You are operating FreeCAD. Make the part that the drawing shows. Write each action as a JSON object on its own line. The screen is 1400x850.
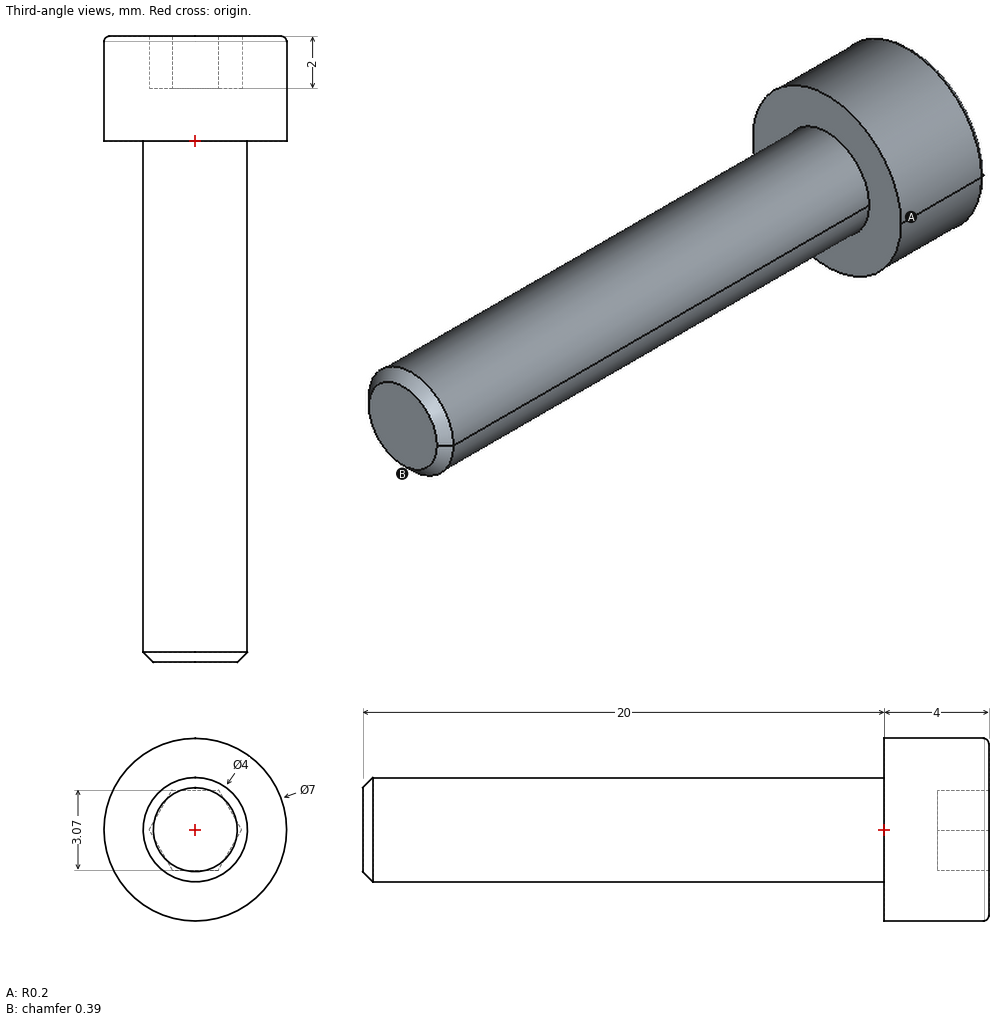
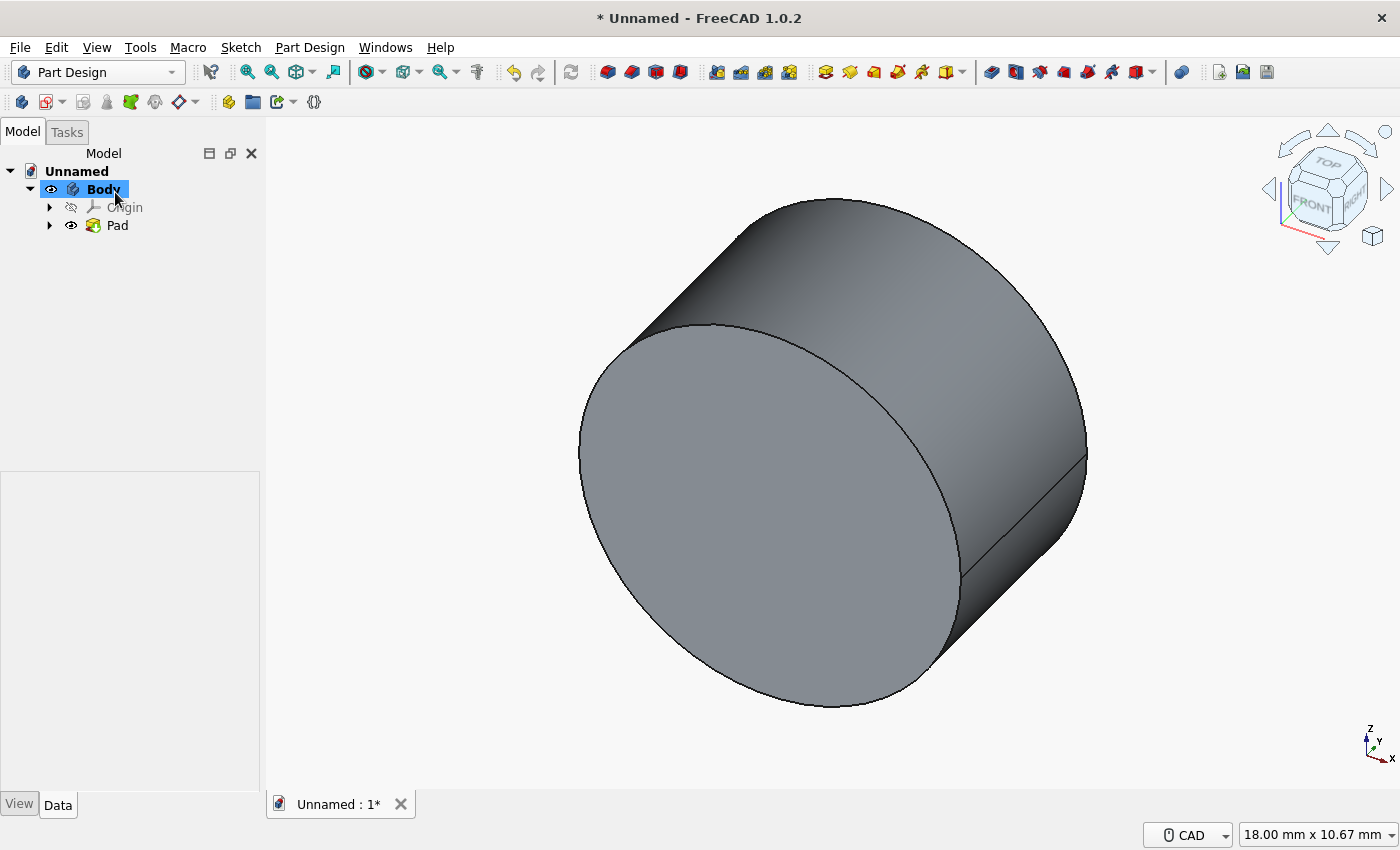
{"action": "key", "text": "4"}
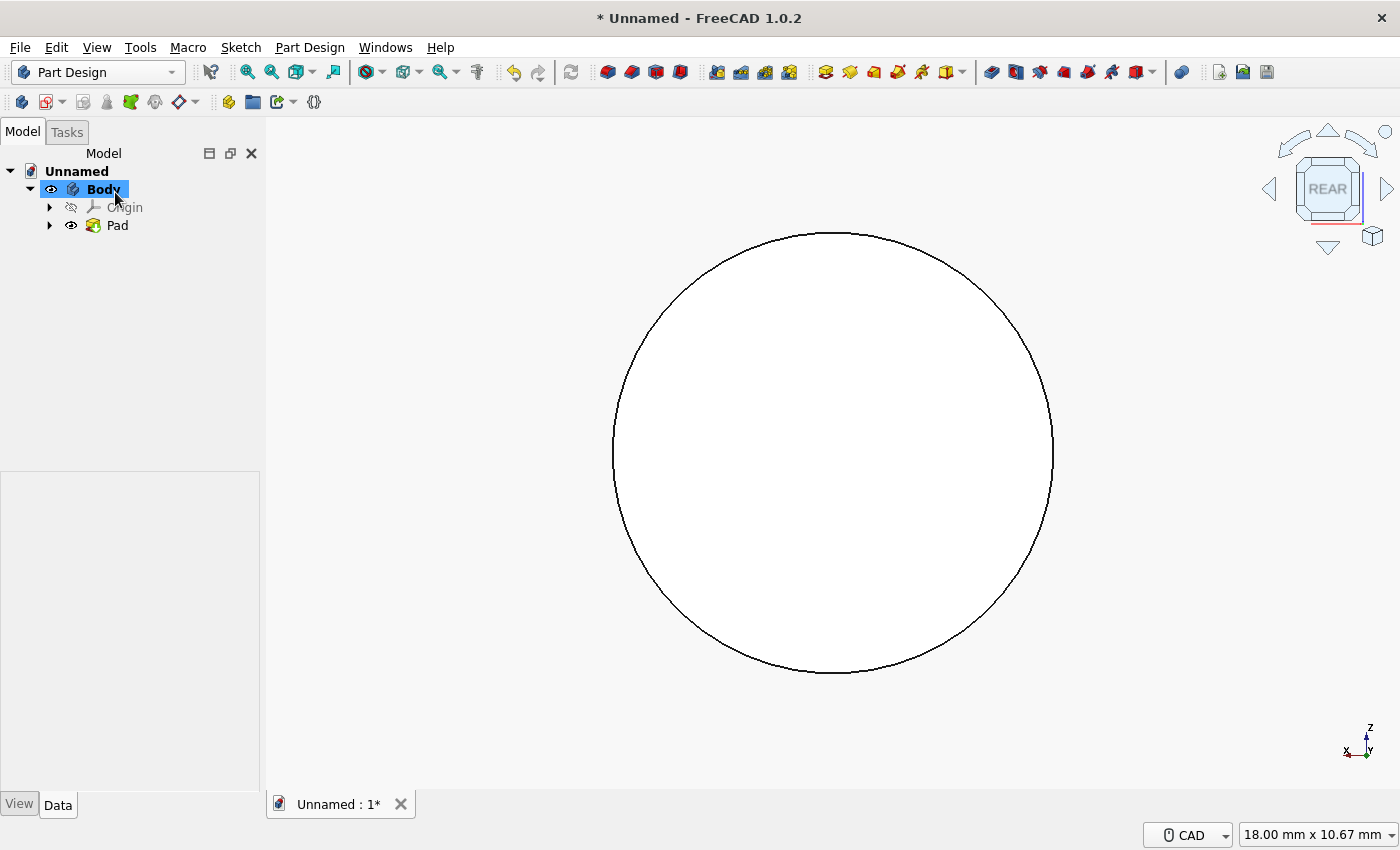
{"action": "left_click", "coordinate": [833, 452]}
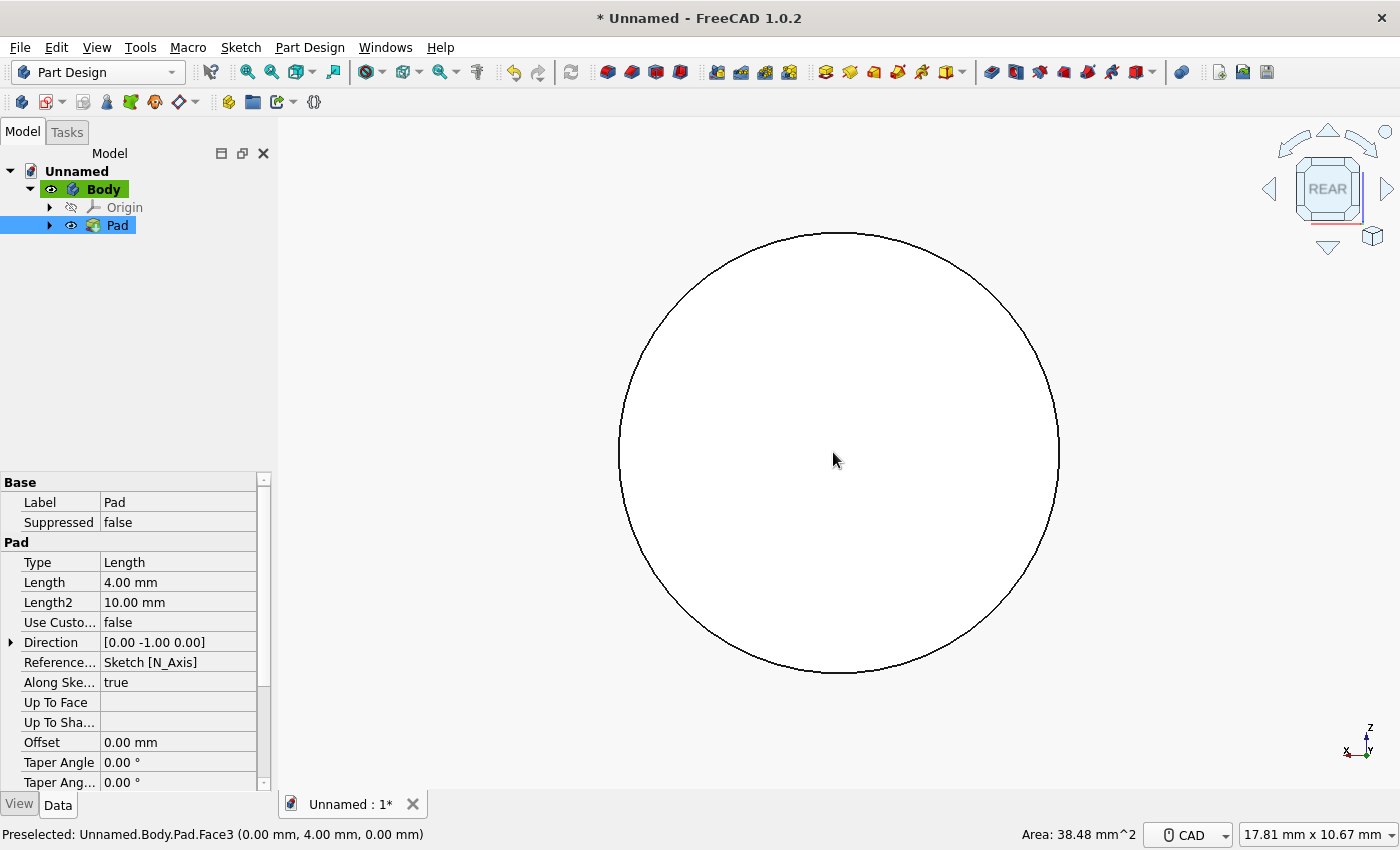
{"action": "left_click", "coordinate": [46, 102]}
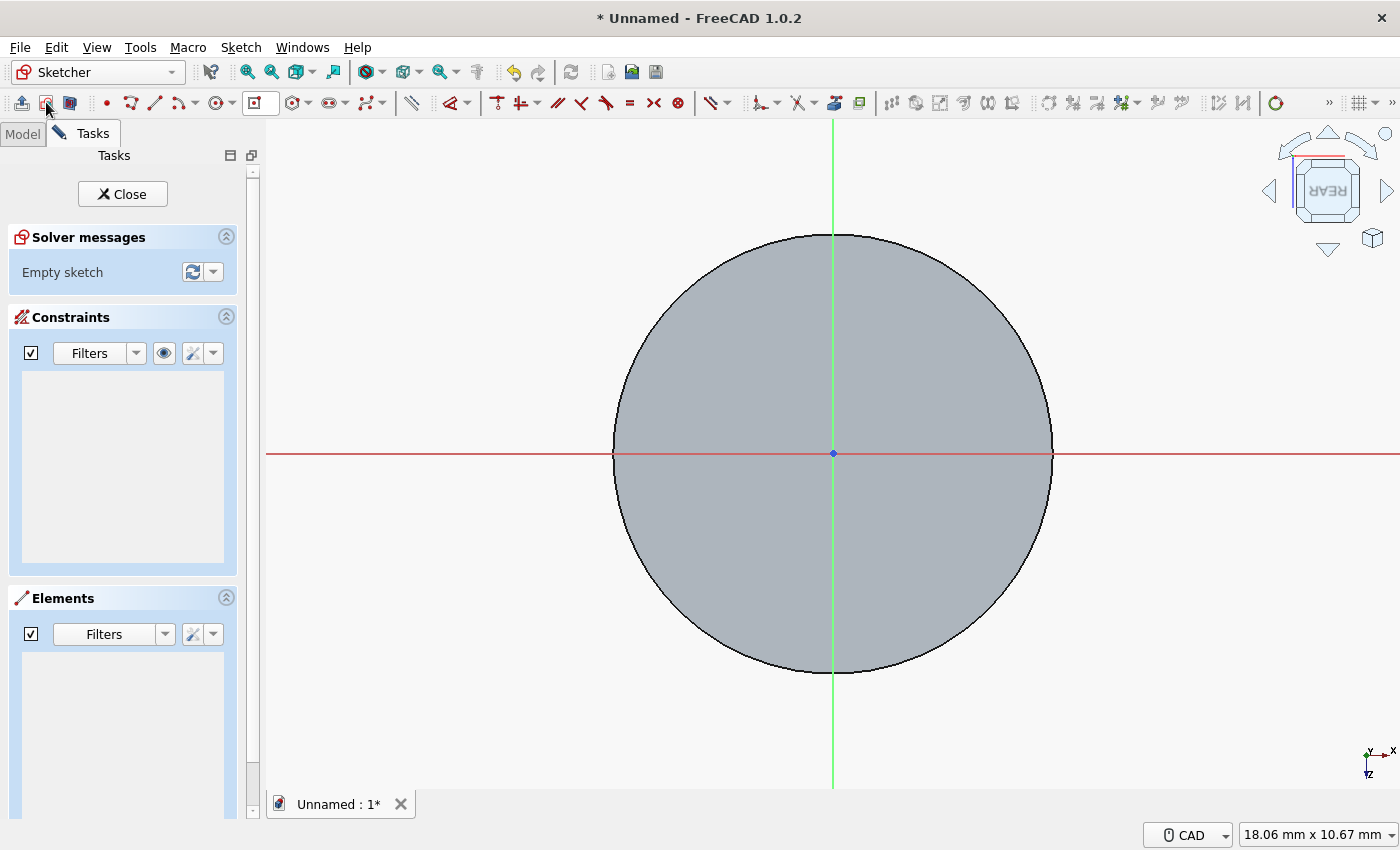
{"action": "scroll", "coordinate": [889, 454], "scroll_direction": "up", "scroll_amount": 4}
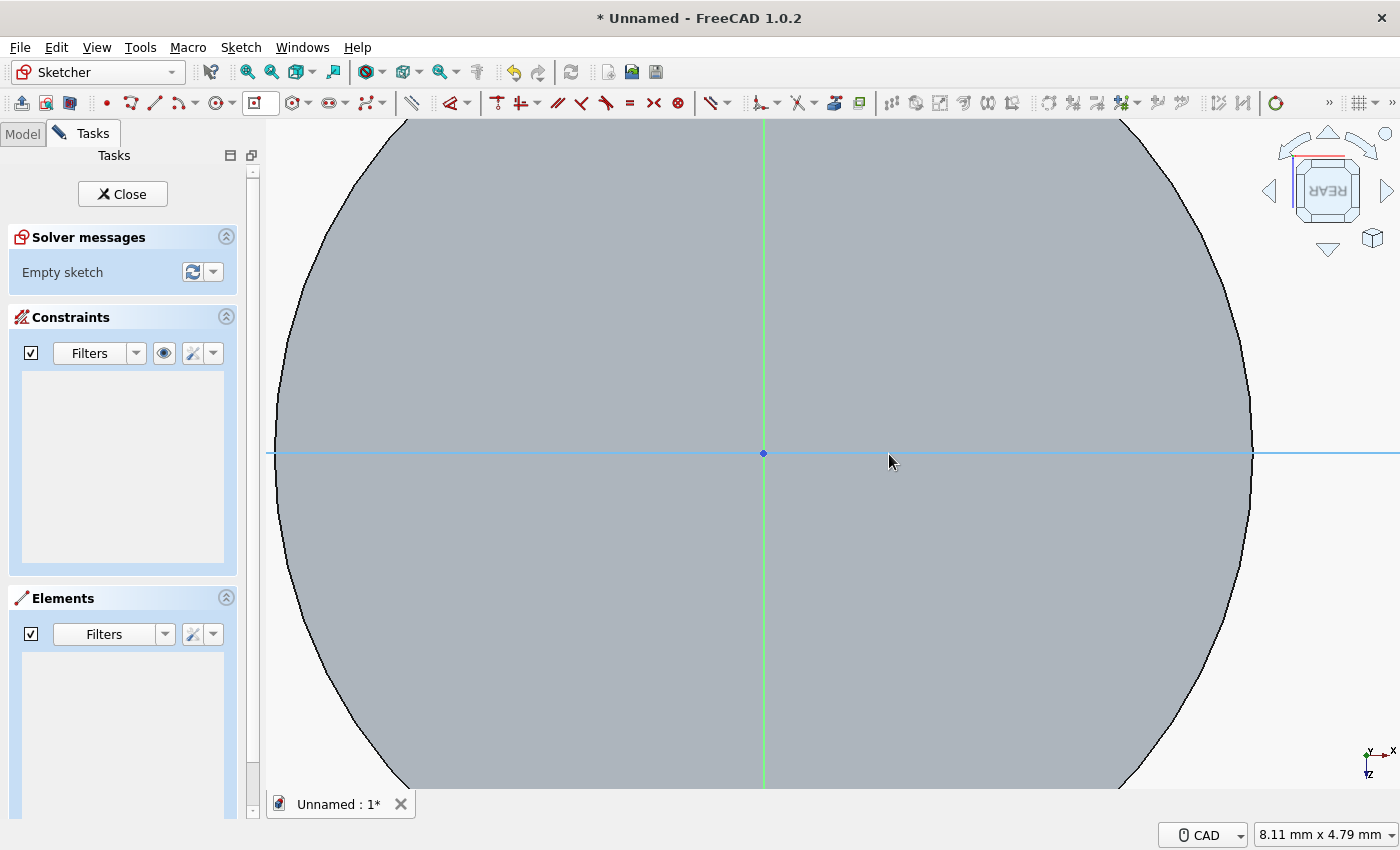
{"action": "key", "text": "g p 6"}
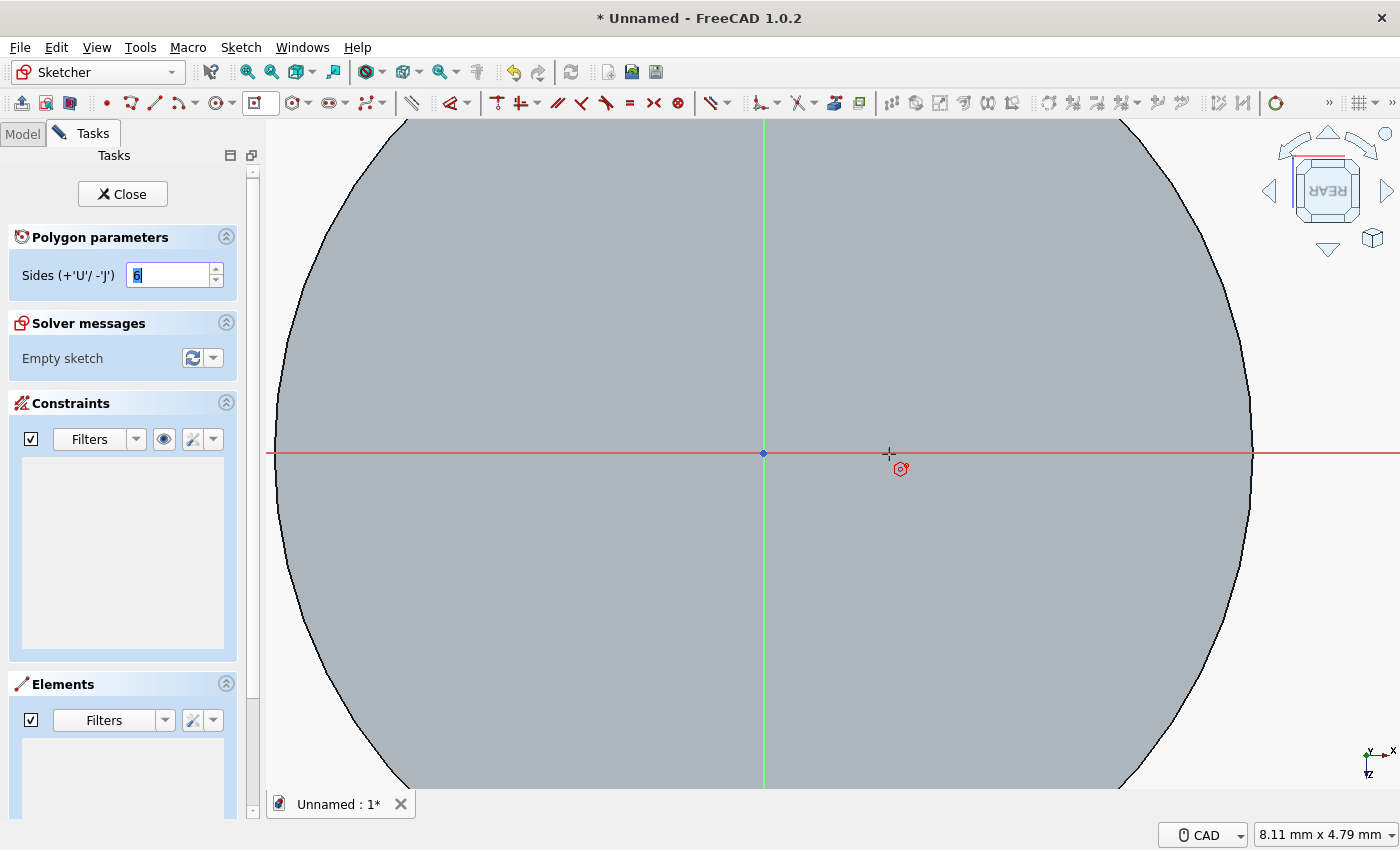
{"action": "left_click", "coordinate": [764, 453]}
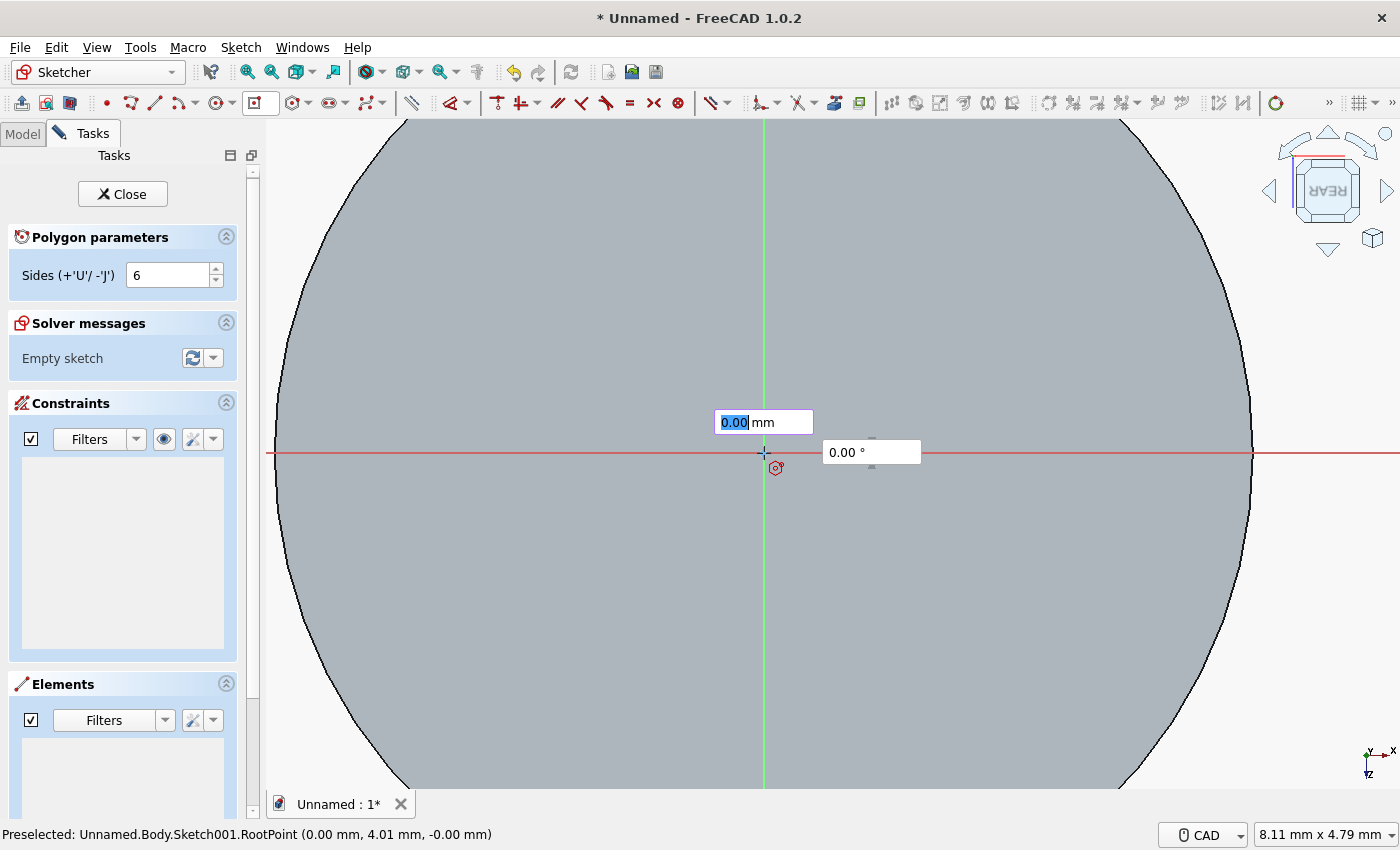
{"action": "left_click", "coordinate": [1011, 453]}
{"action": "right_click", "coordinate": [1011, 453]}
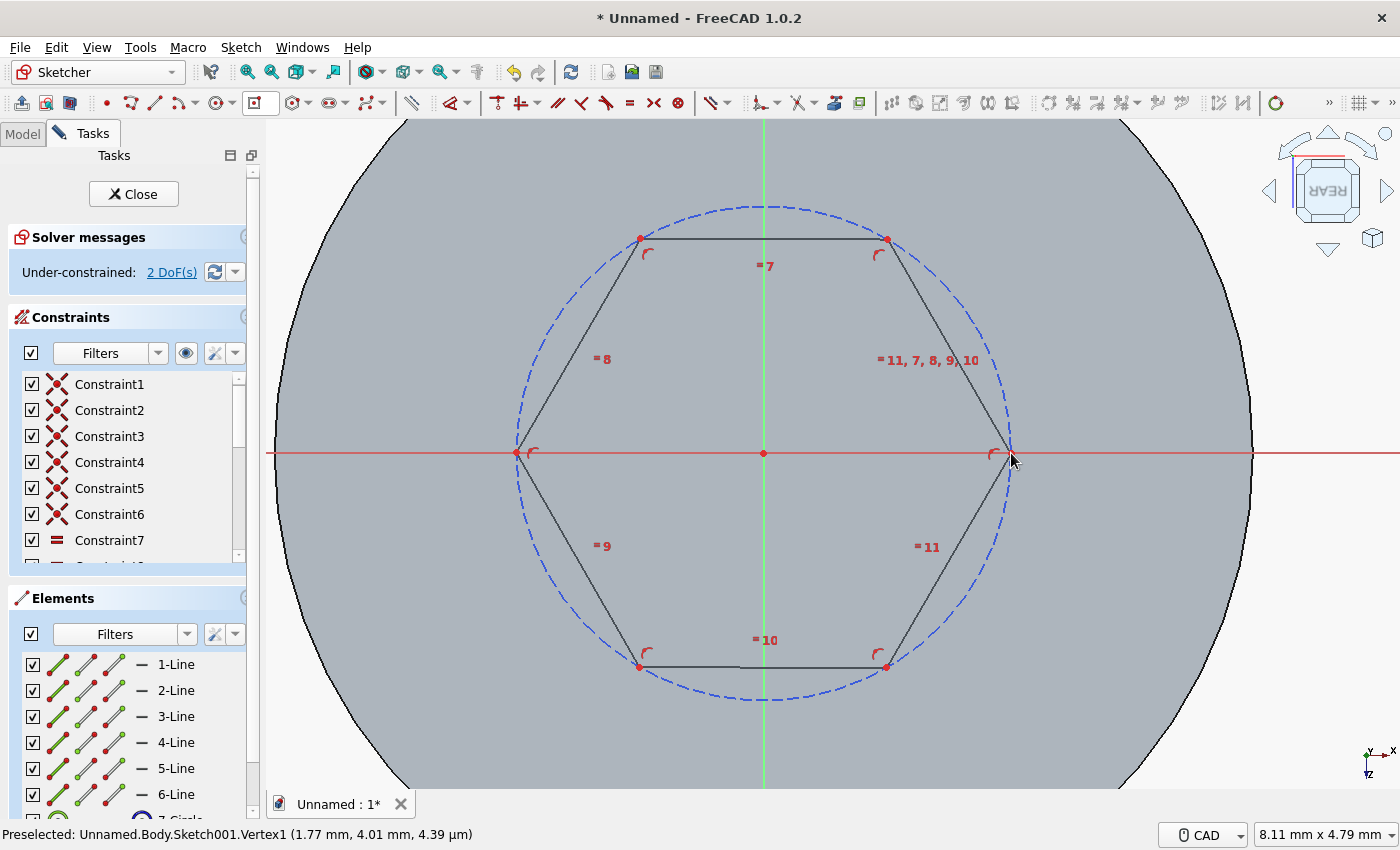
{"action": "left_click", "coordinate": [814, 239]}